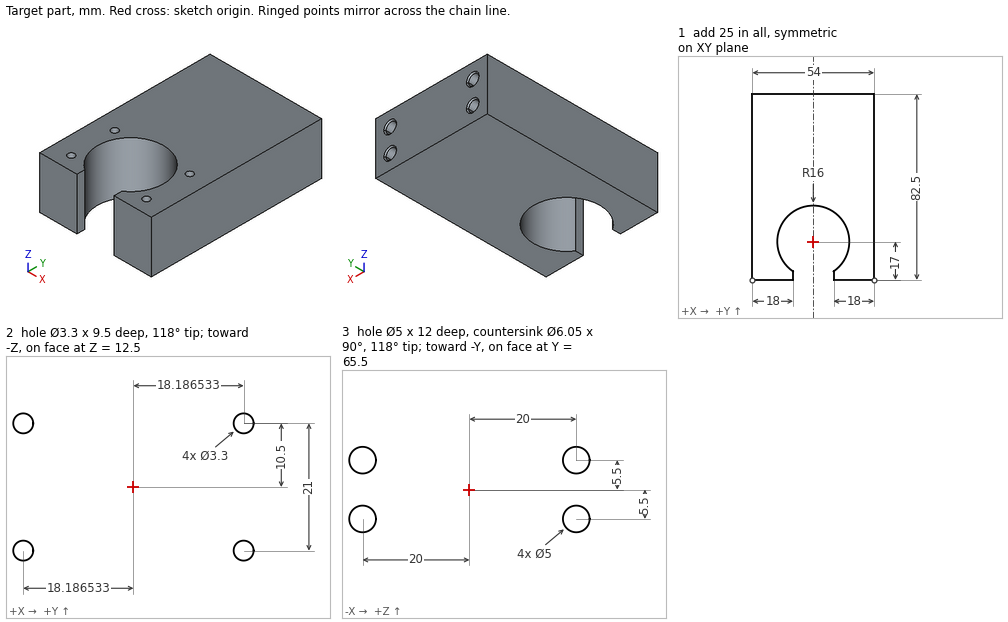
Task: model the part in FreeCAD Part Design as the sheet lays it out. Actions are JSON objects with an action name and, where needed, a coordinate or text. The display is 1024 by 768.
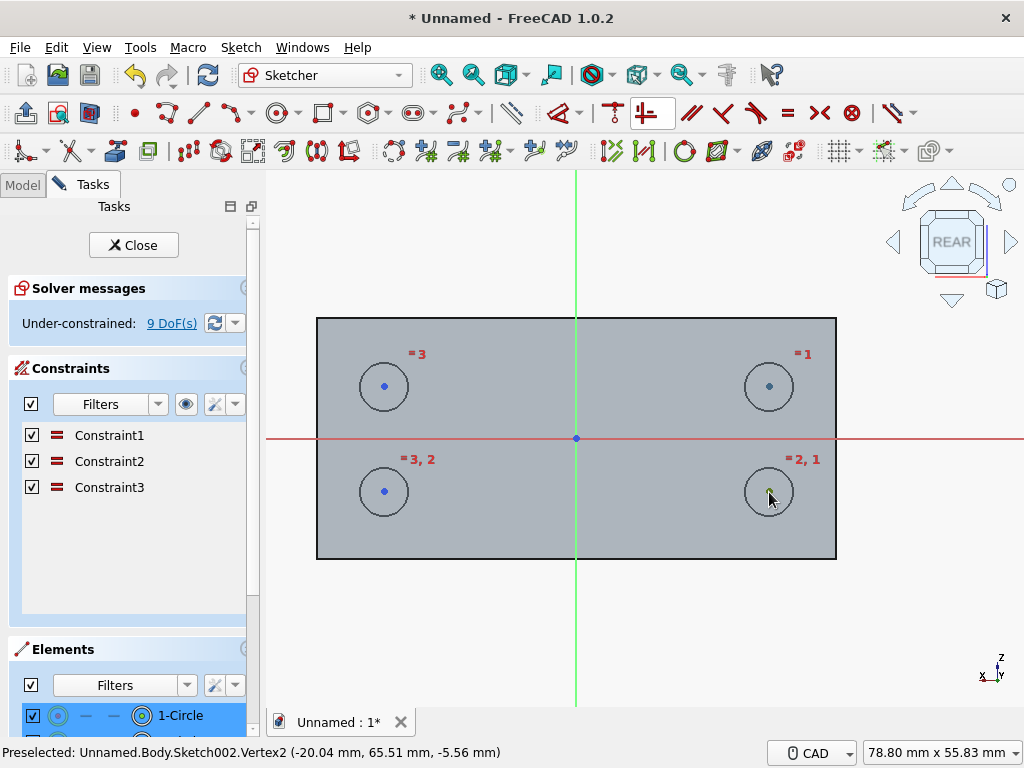
{"action": "left_click", "coordinate": [670, 114]}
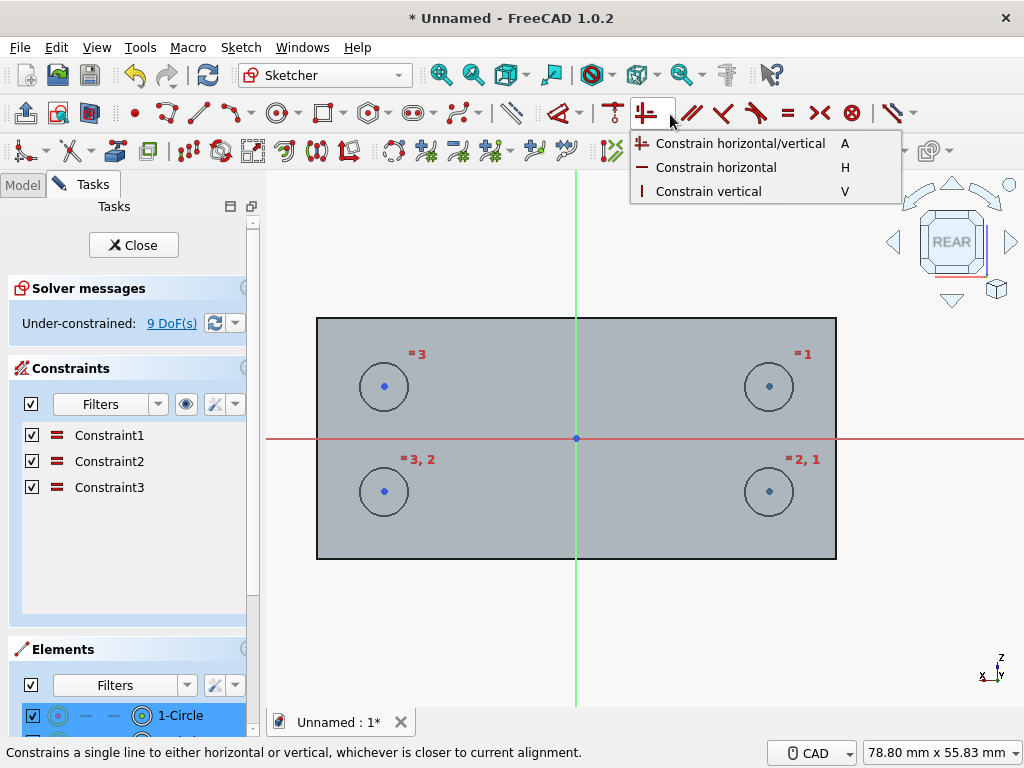
{"action": "left_click", "coordinate": [766, 191]}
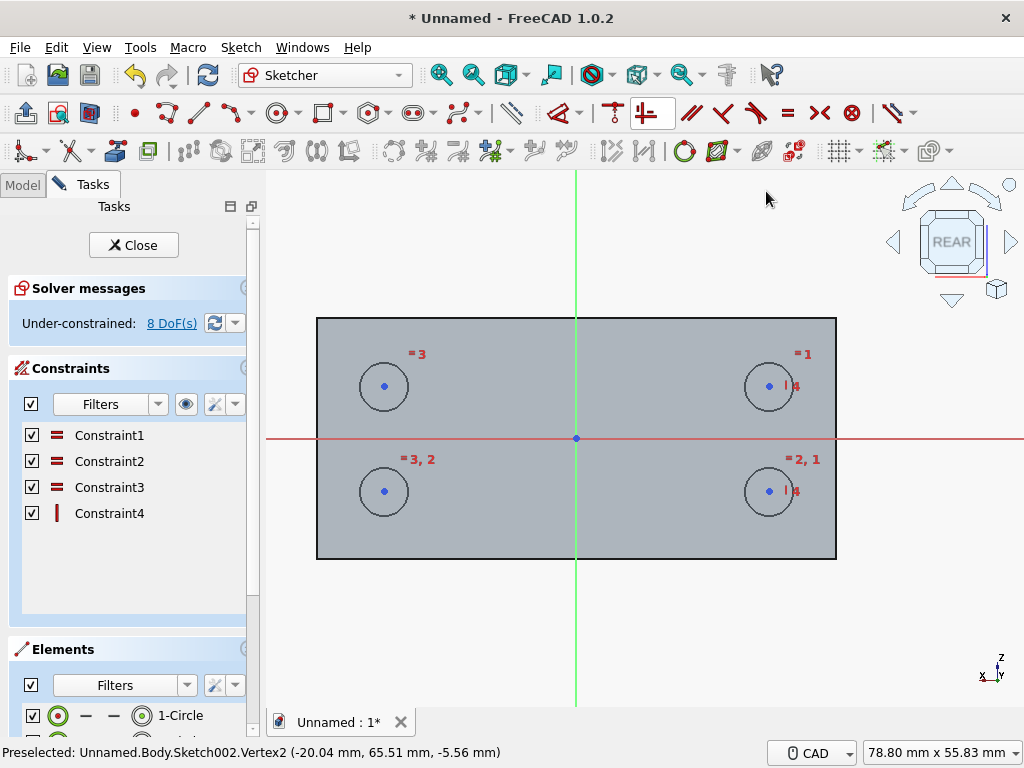
{"action": "left_click", "coordinate": [769, 492]}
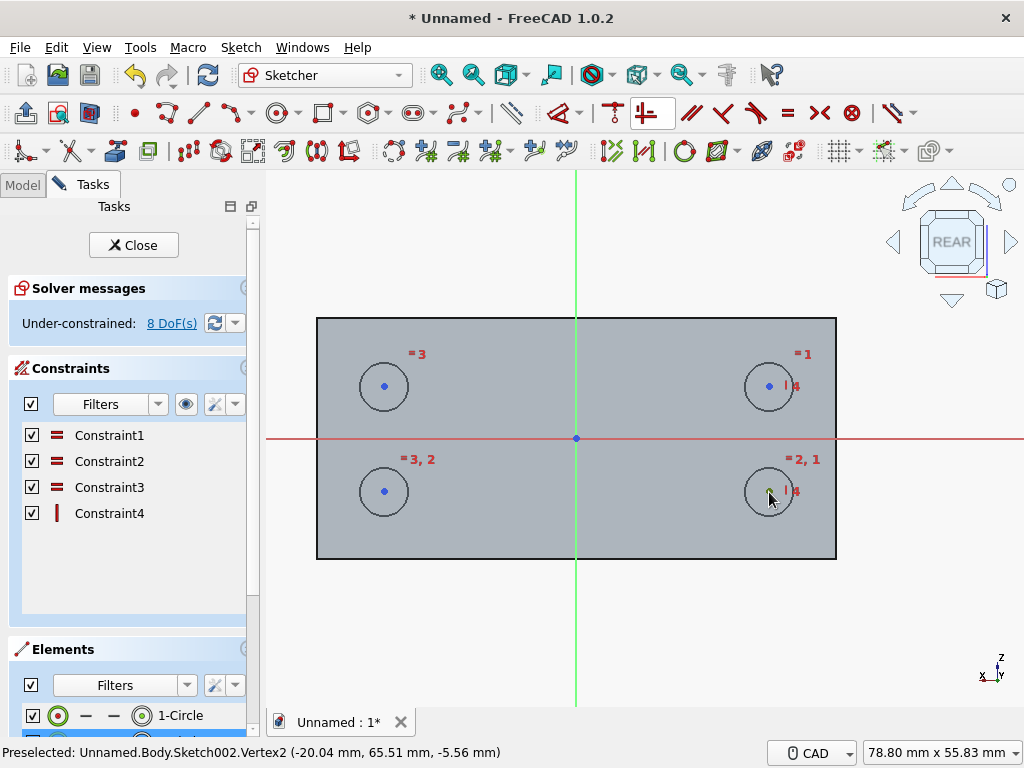
{"action": "left_click", "coordinate": [384, 492]}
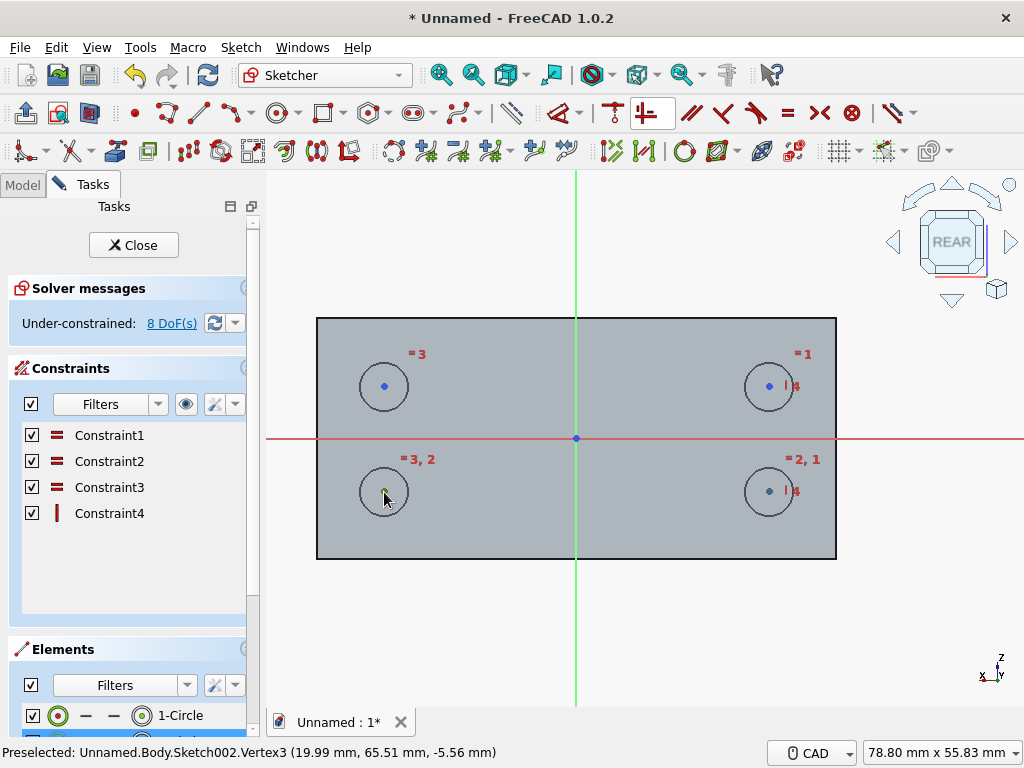
{"action": "left_click", "coordinate": [670, 114]}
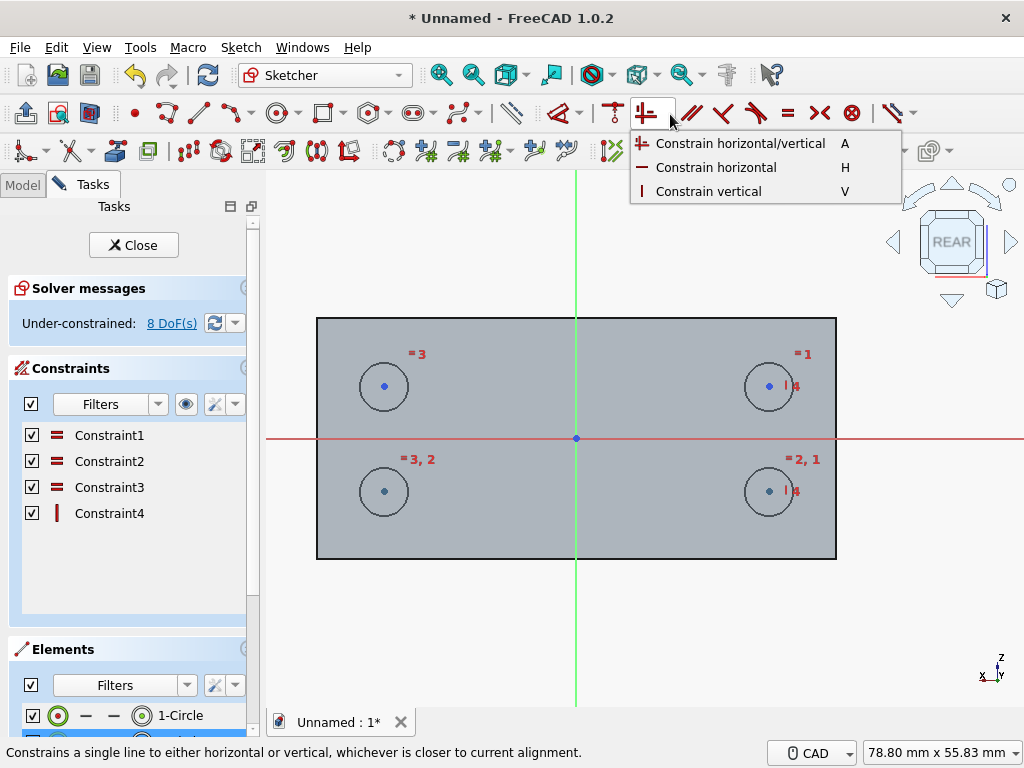
{"action": "left_click", "coordinate": [766, 167]}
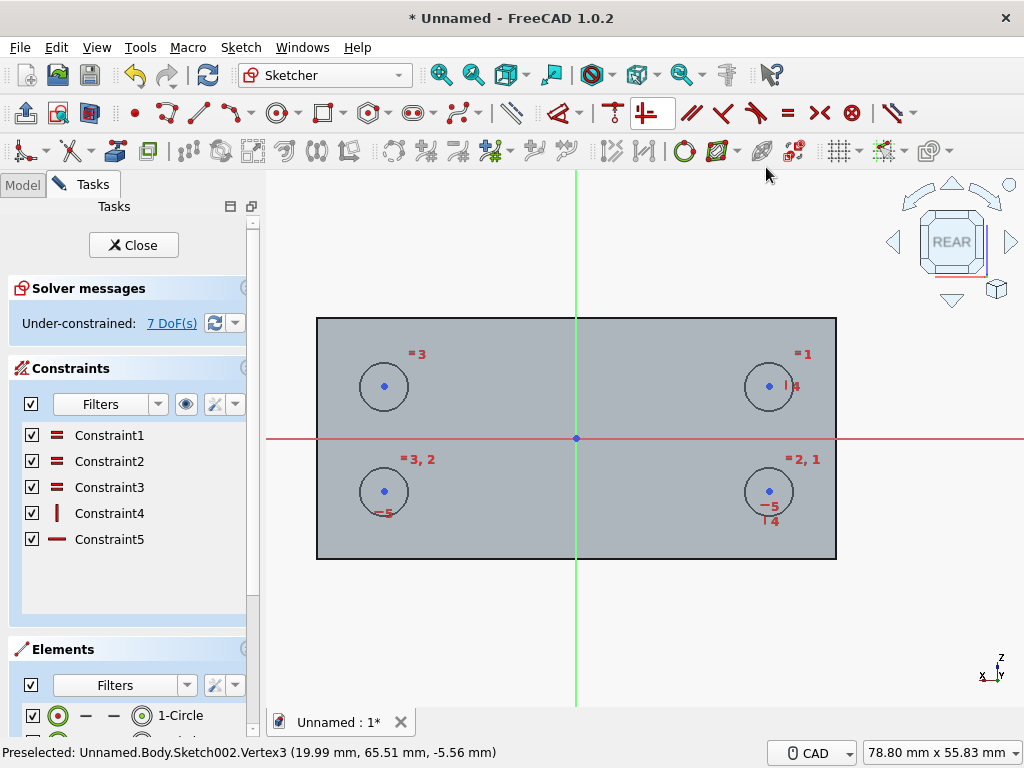
{"action": "left_click", "coordinate": [384, 492]}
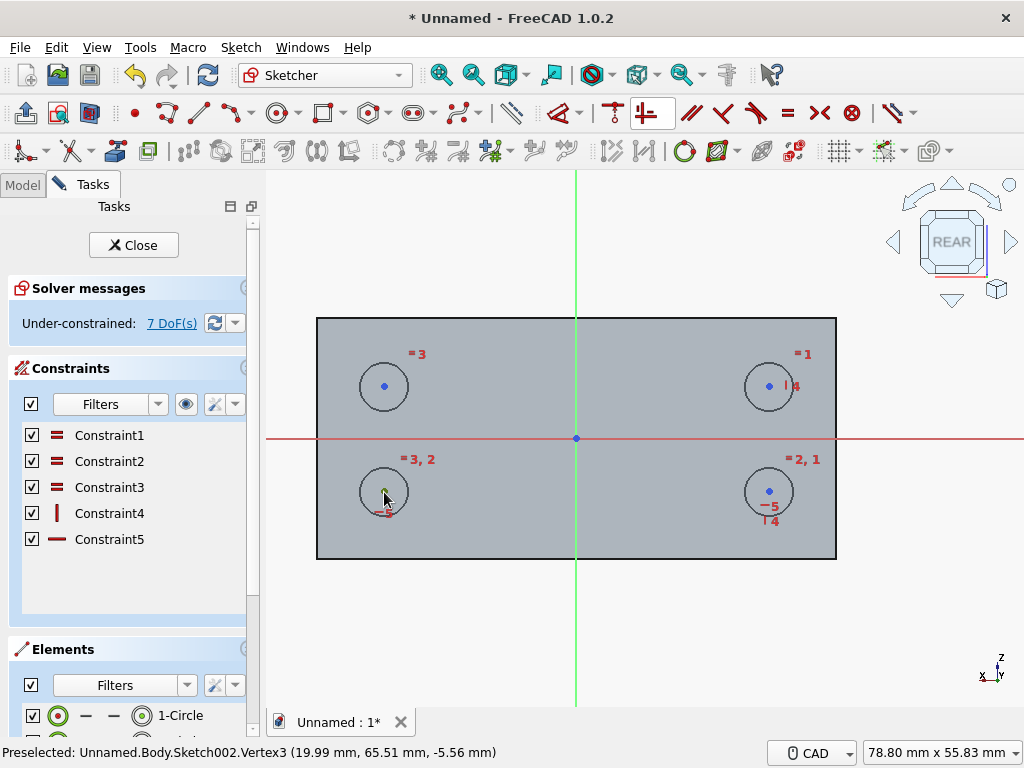
{"action": "left_click", "coordinate": [384, 387]}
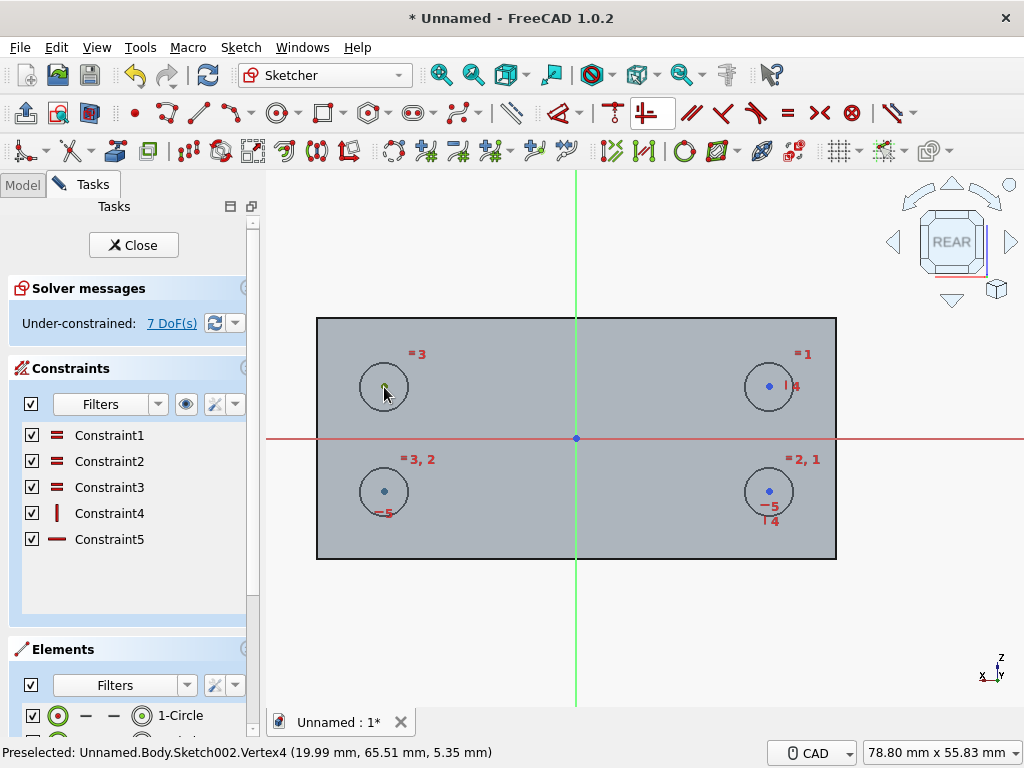
{"action": "key", "text": "v"}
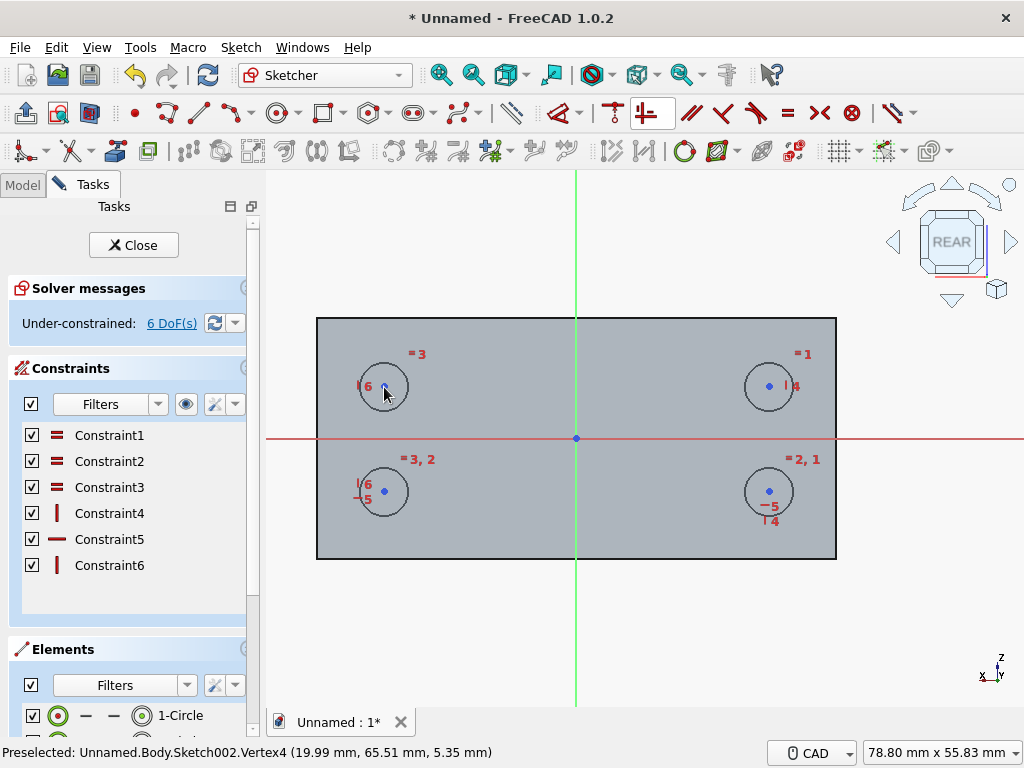
{"action": "left_click", "coordinate": [769, 387]}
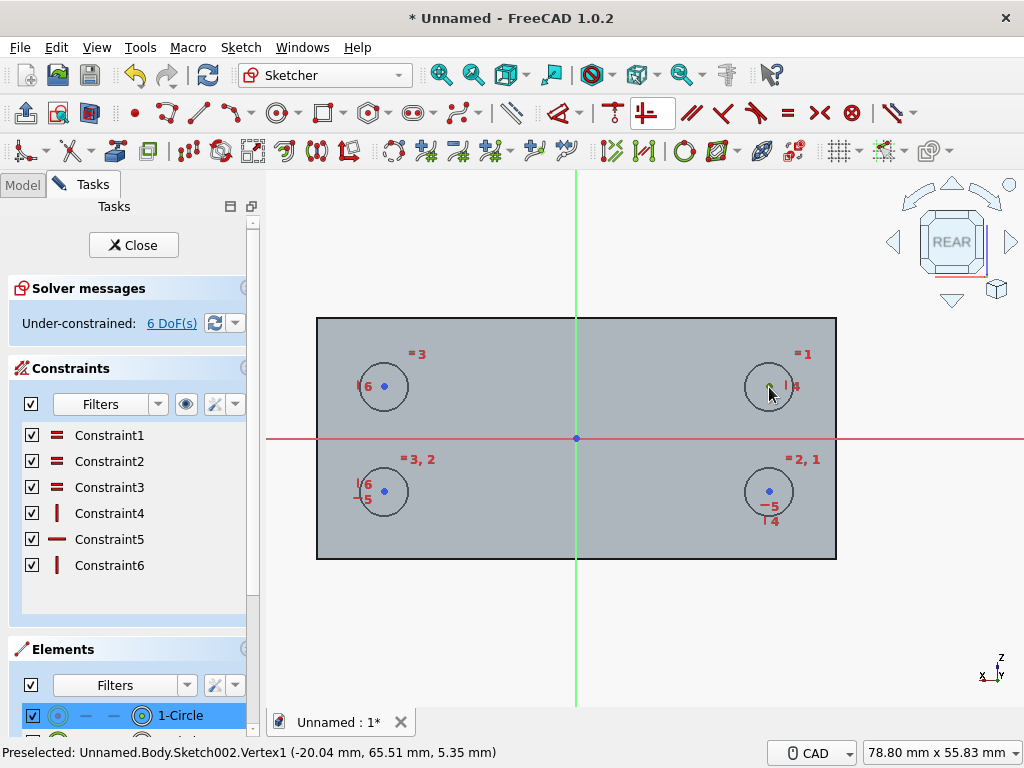
{"action": "left_click", "coordinate": [384, 387]}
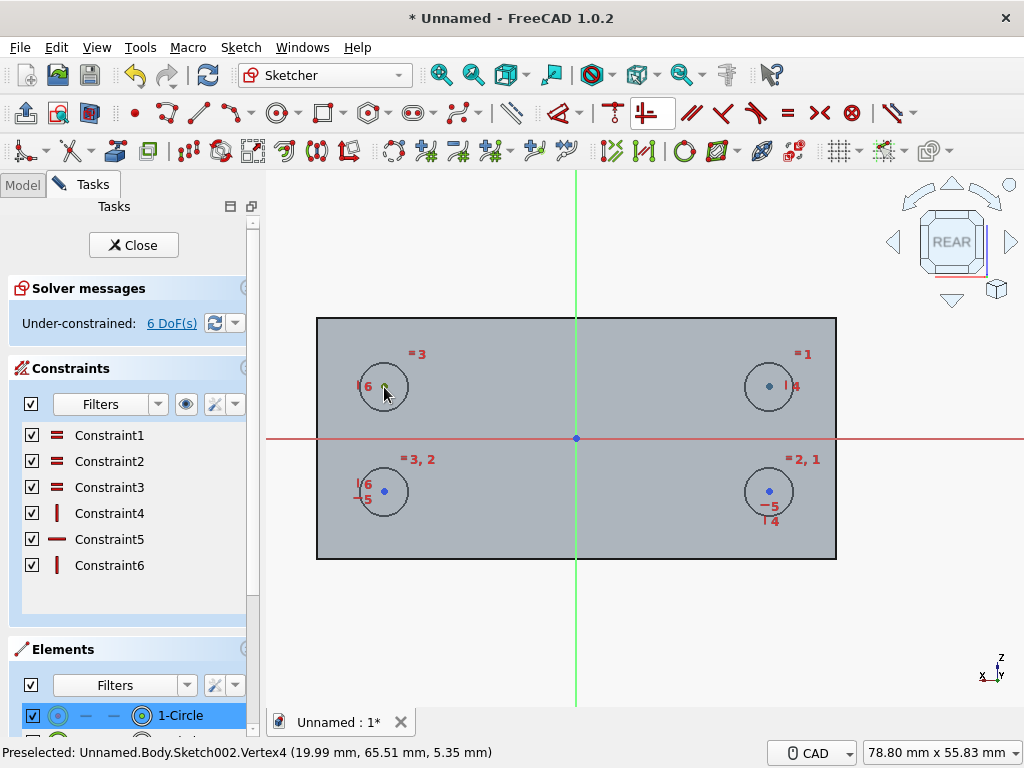
{"action": "key", "text": "h"}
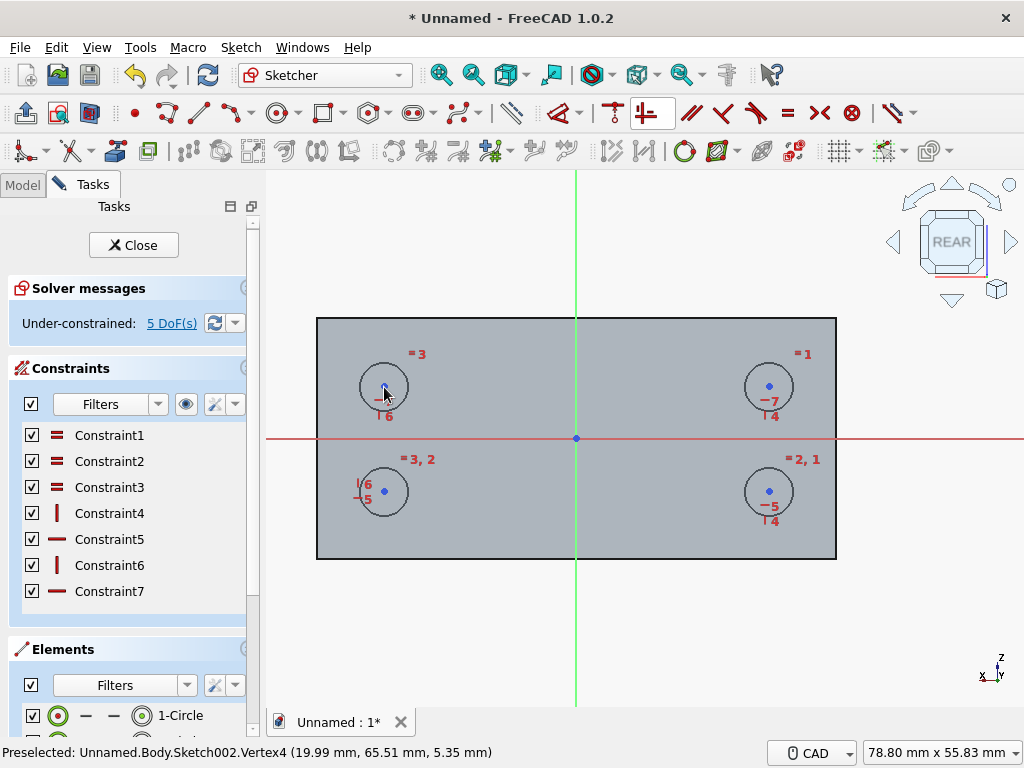
{"action": "left_click", "coordinate": [558, 114]}